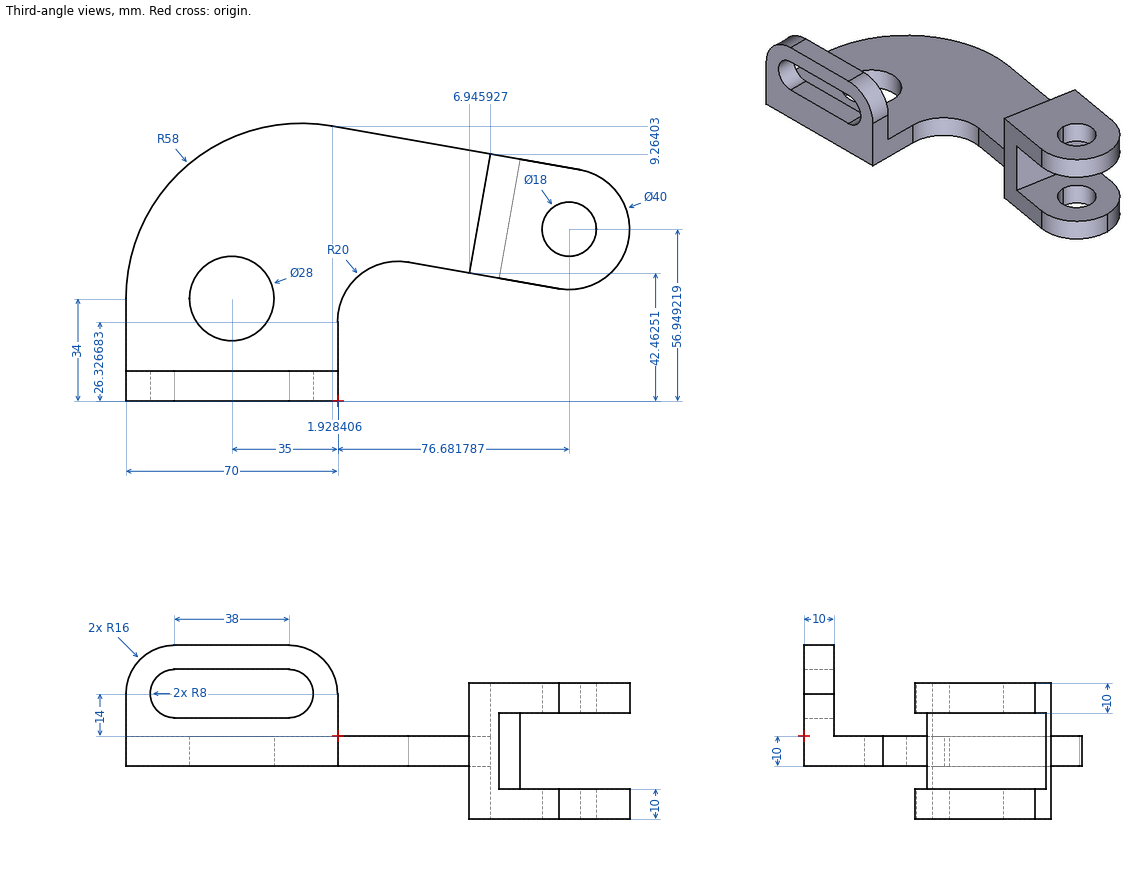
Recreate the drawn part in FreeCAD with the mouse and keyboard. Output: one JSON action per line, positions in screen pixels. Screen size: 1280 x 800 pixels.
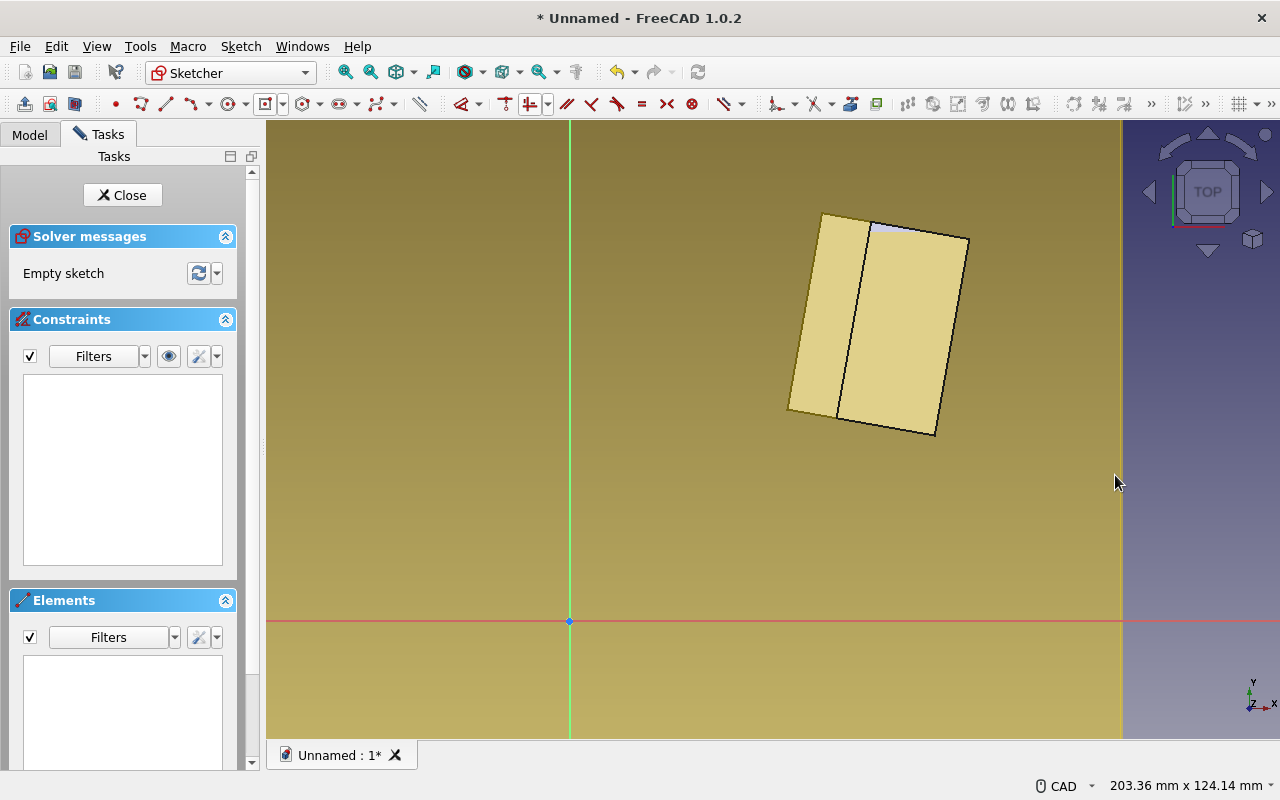
{"action": "left_click", "coordinate": [228, 104]}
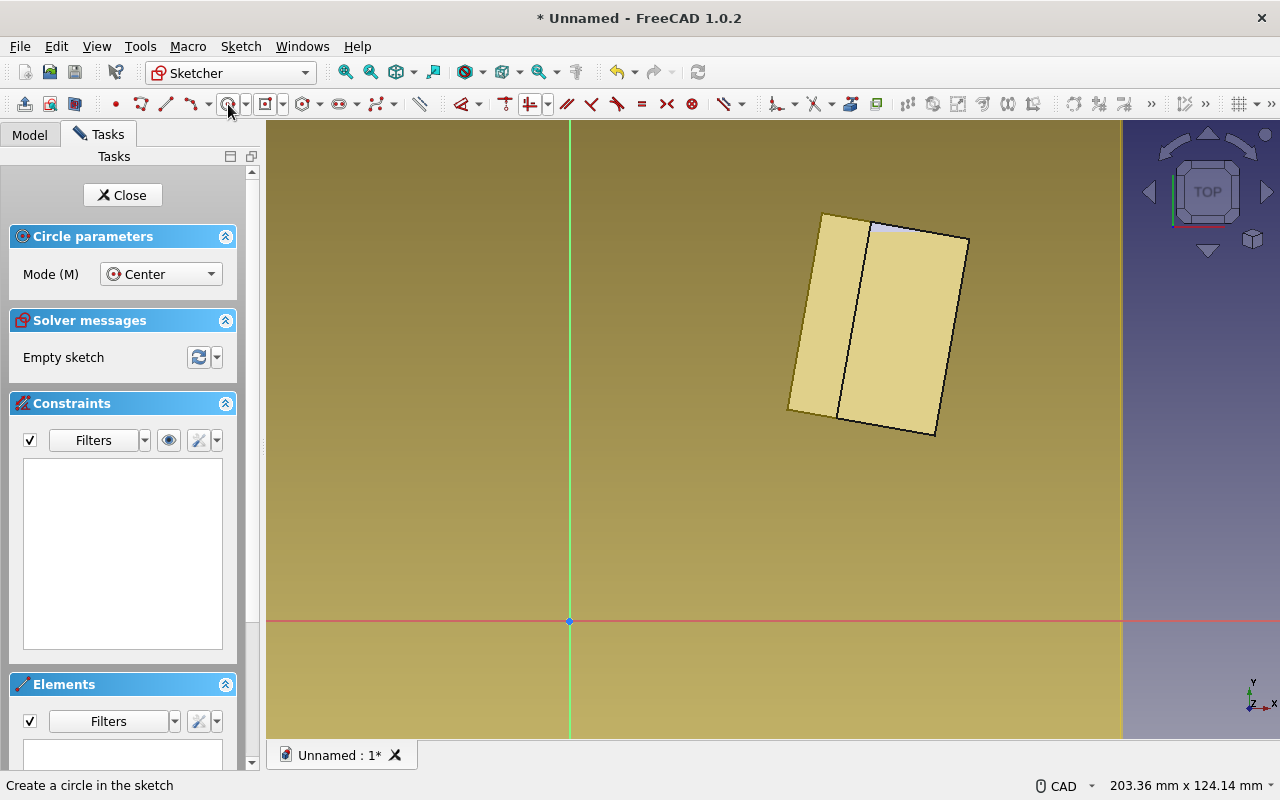
{"action": "left_click", "coordinate": [952, 337]}
{"action": "left_click", "coordinate": [1023, 267]}
{"action": "key", "text": "Escape"}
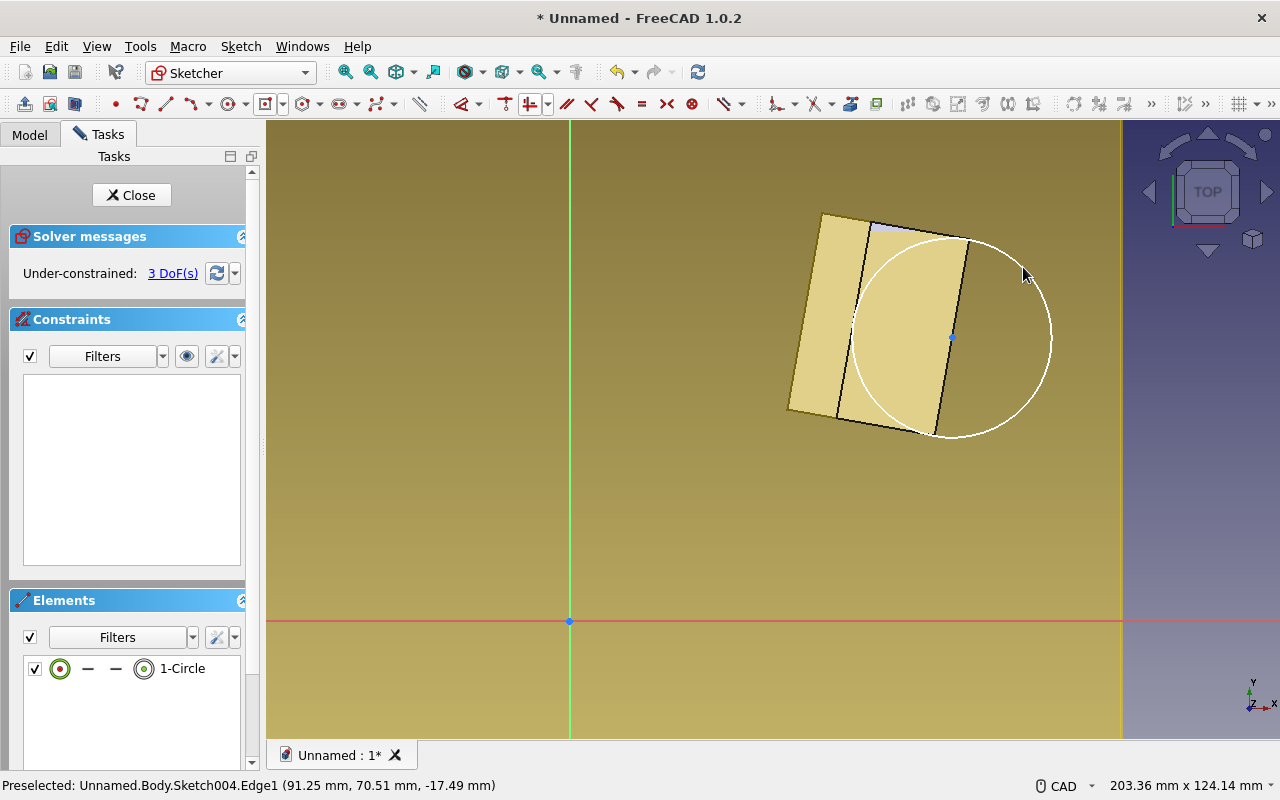
{"action": "left_click", "coordinate": [460, 104]}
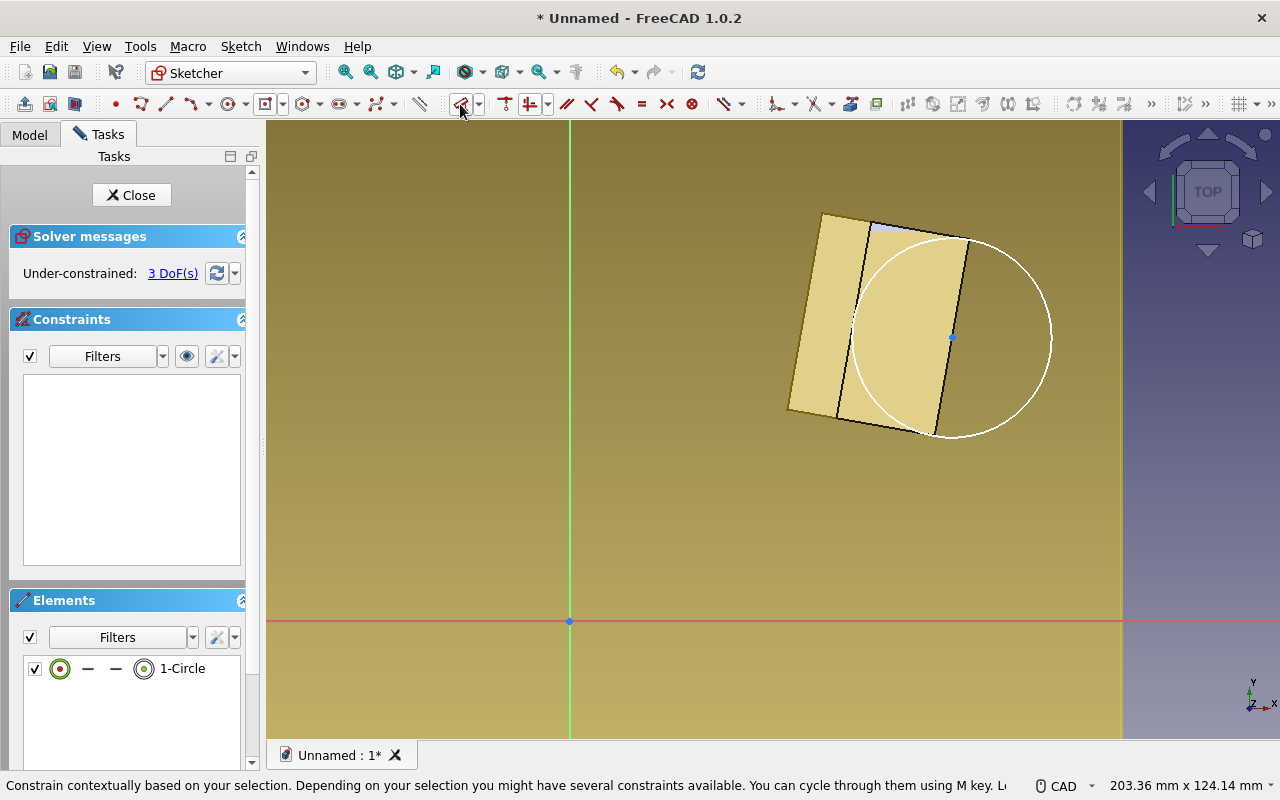
{"action": "left_click", "coordinate": [1022, 267]}
{"action": "left_click", "coordinate": [1044, 244]}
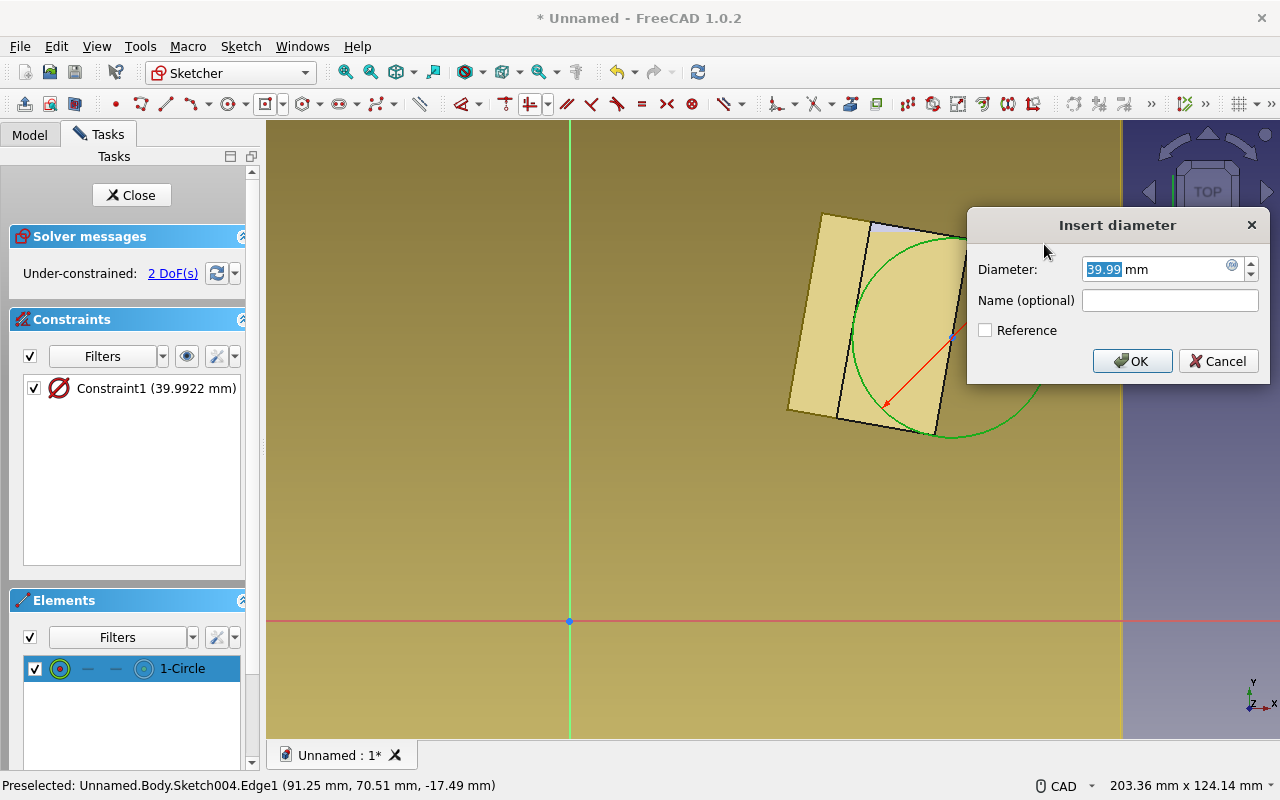
{"action": "type", "text": "40"}
{"action": "key", "text": "Return"}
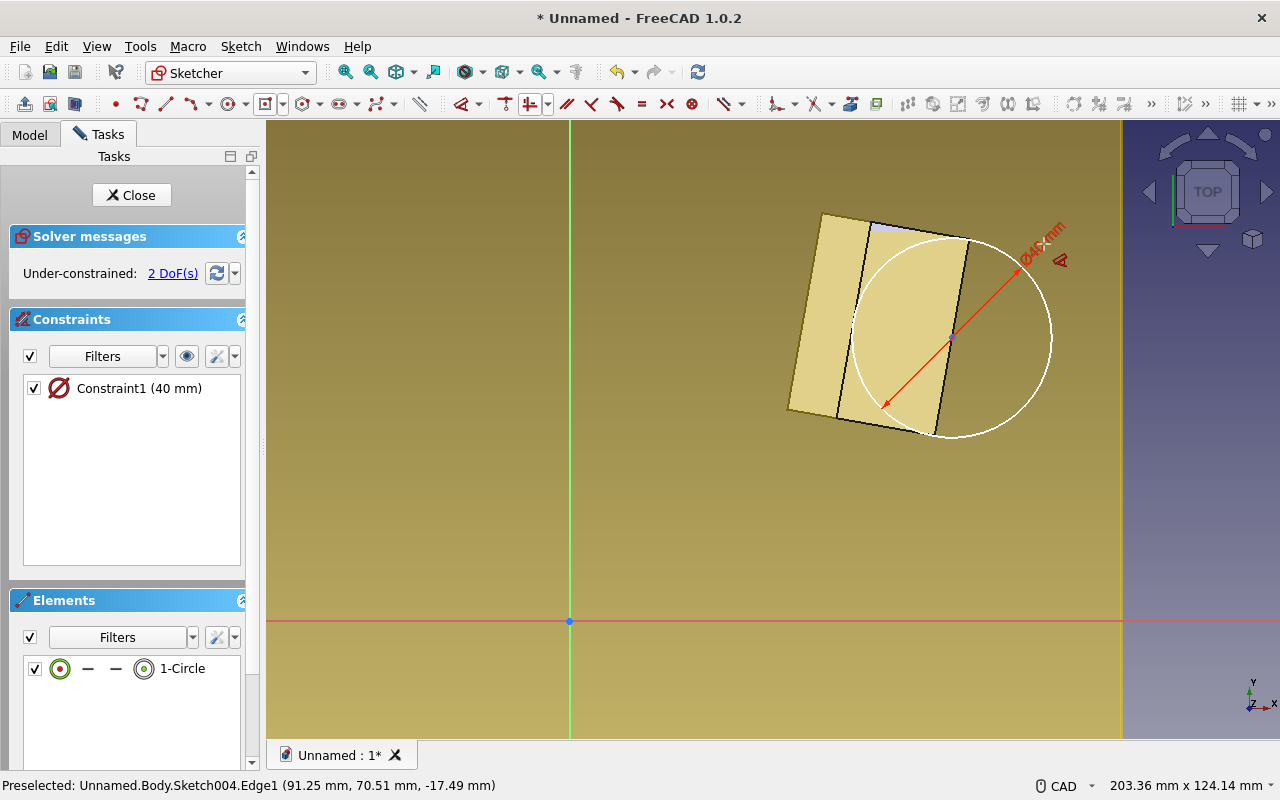
{"action": "left_click", "coordinate": [952, 338]}
{"action": "left_click", "coordinate": [761, 655]}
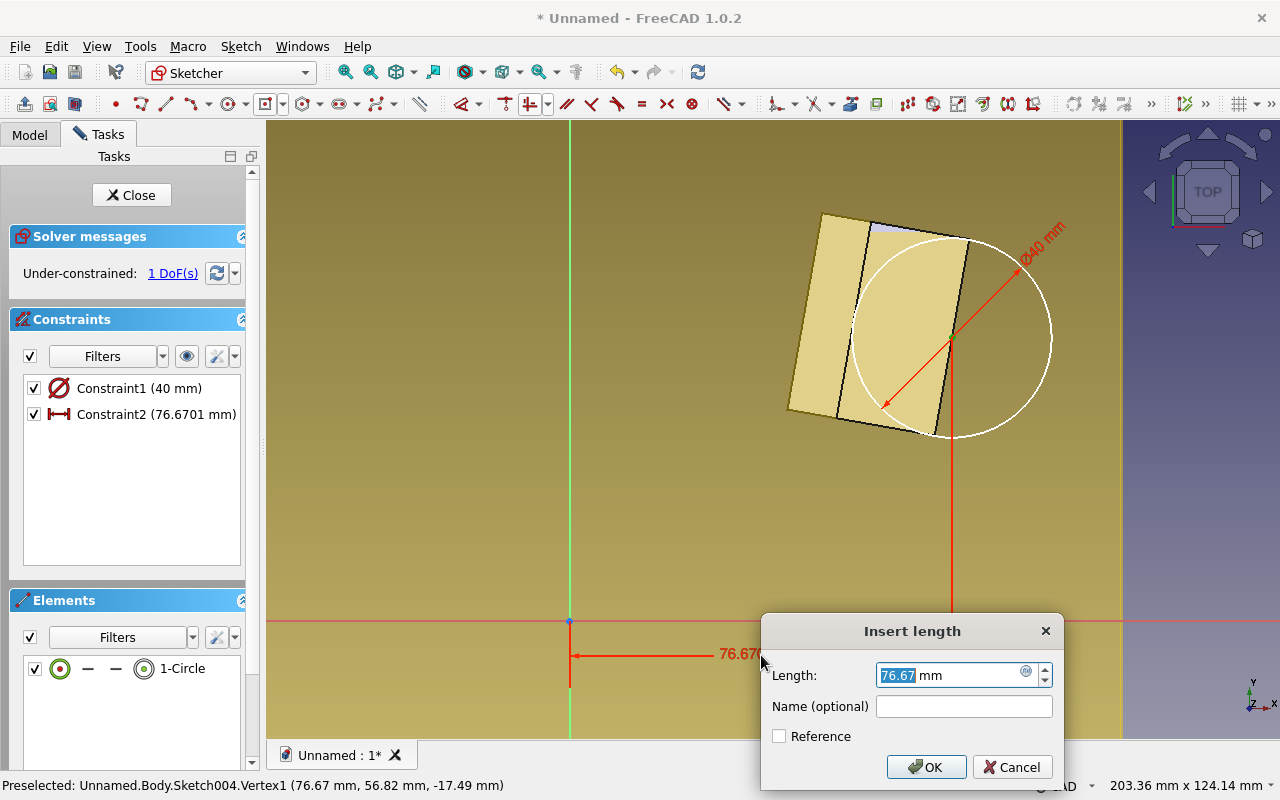
{"action": "type", "text": "76.681787"}
{"action": "key", "text": "Return"}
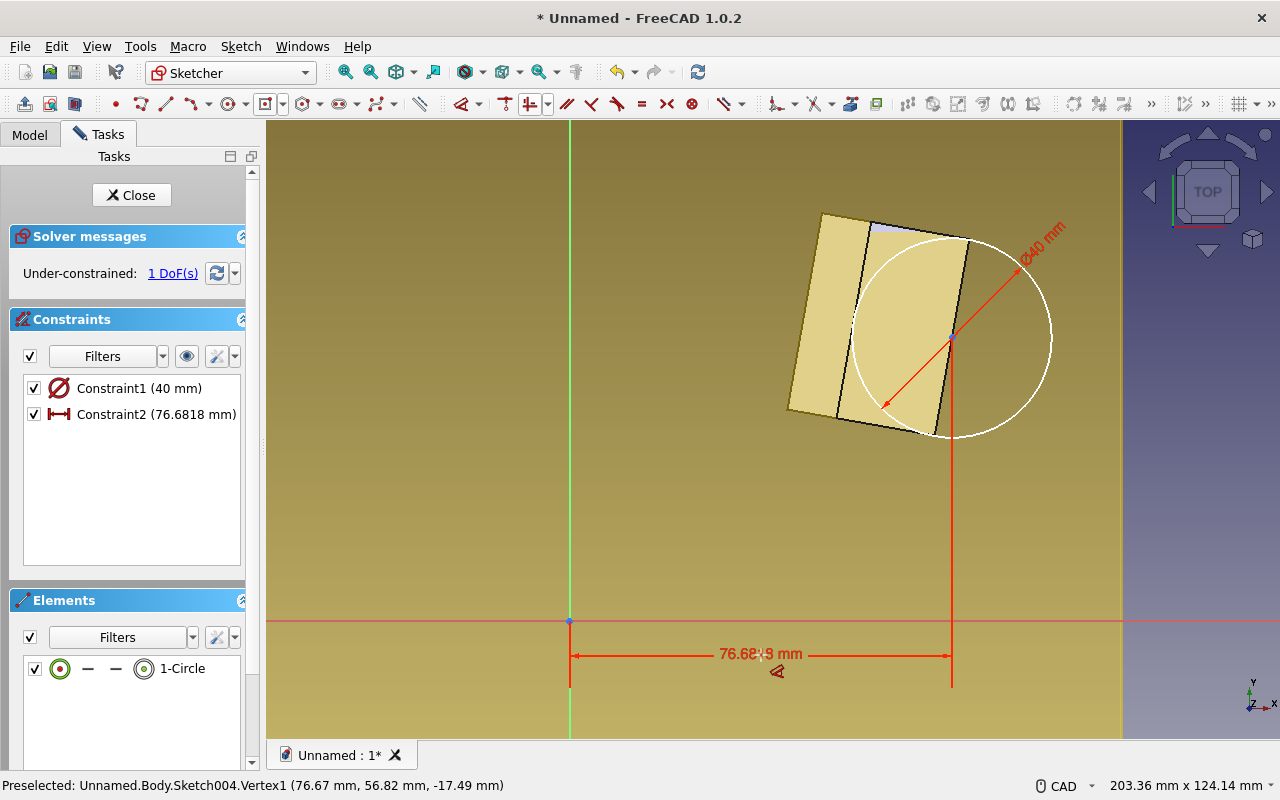
{"action": "left_click", "coordinate": [952, 338]}
{"action": "left_click", "coordinate": [536, 480]}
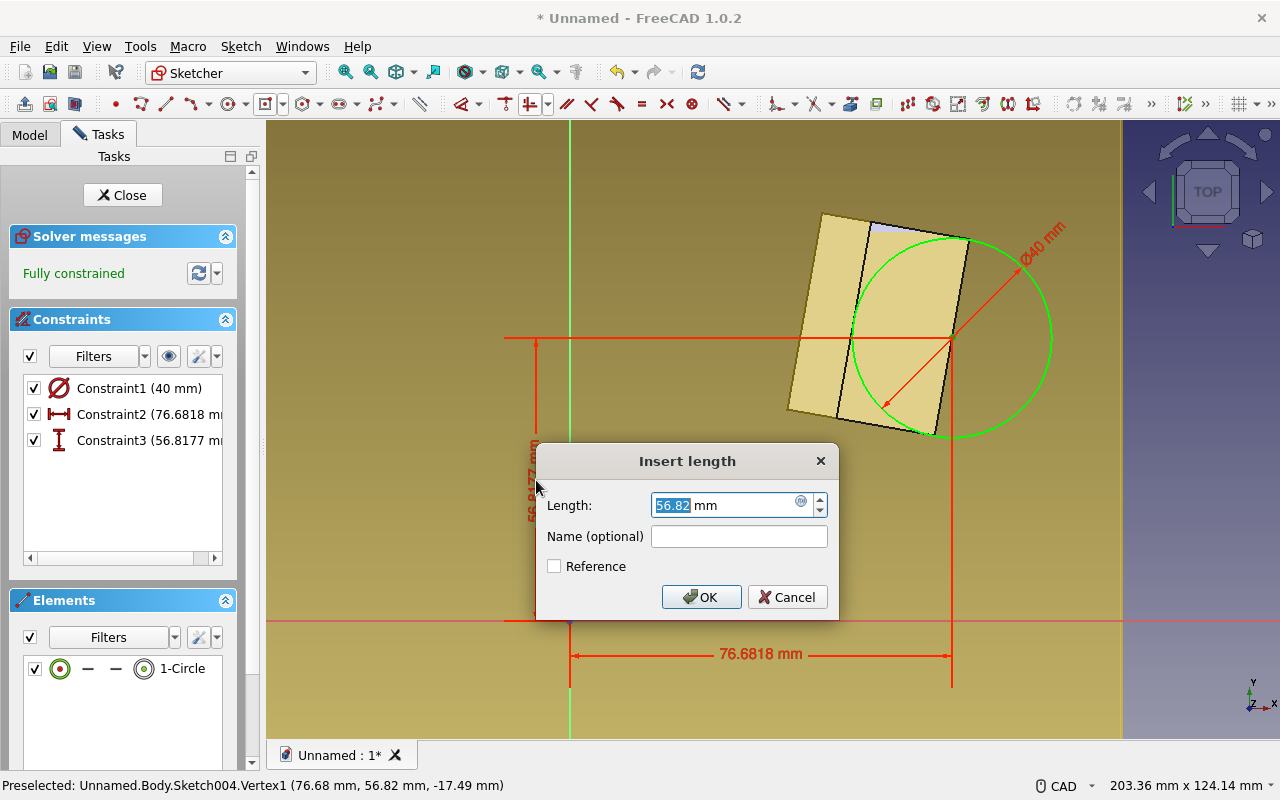
{"action": "type", "text": "56.949219"}
{"action": "key", "text": "Return"}
{"action": "key", "text": "Escape"}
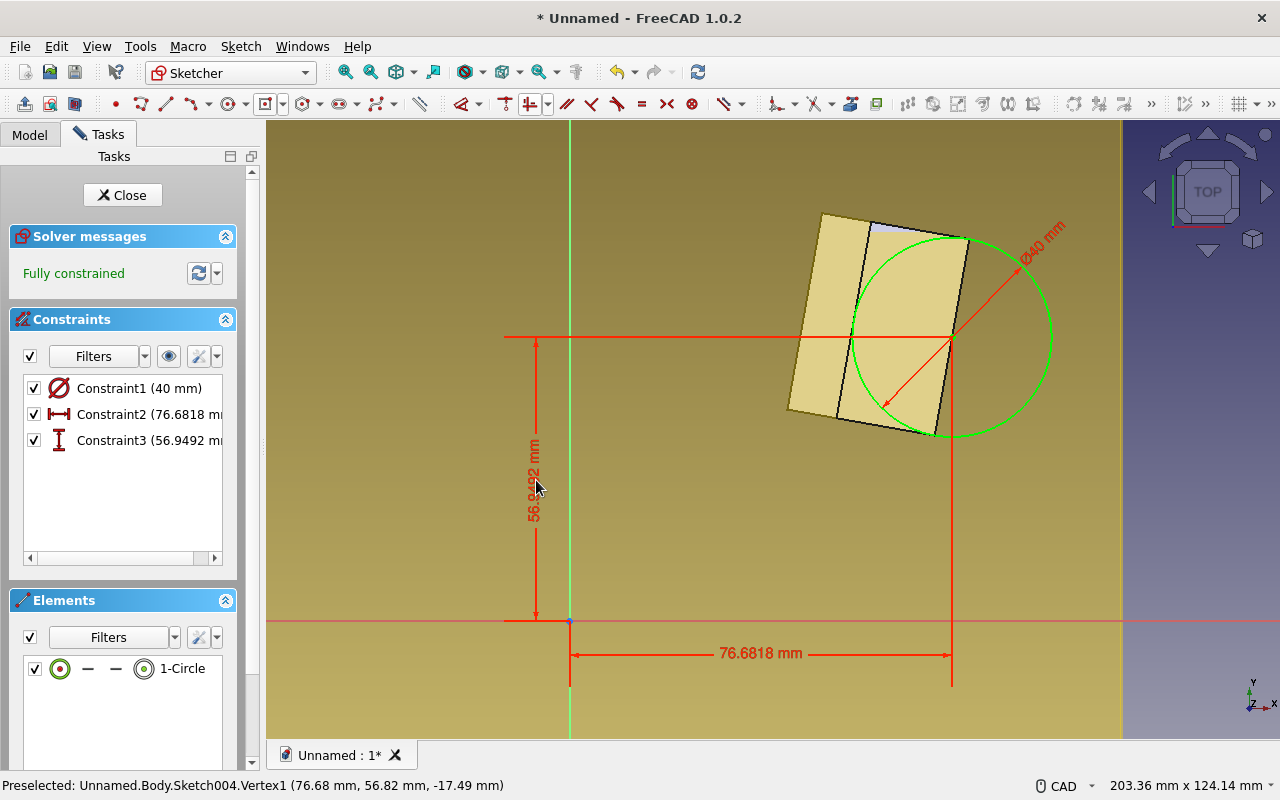
{"action": "left_click", "coordinate": [123, 195]}